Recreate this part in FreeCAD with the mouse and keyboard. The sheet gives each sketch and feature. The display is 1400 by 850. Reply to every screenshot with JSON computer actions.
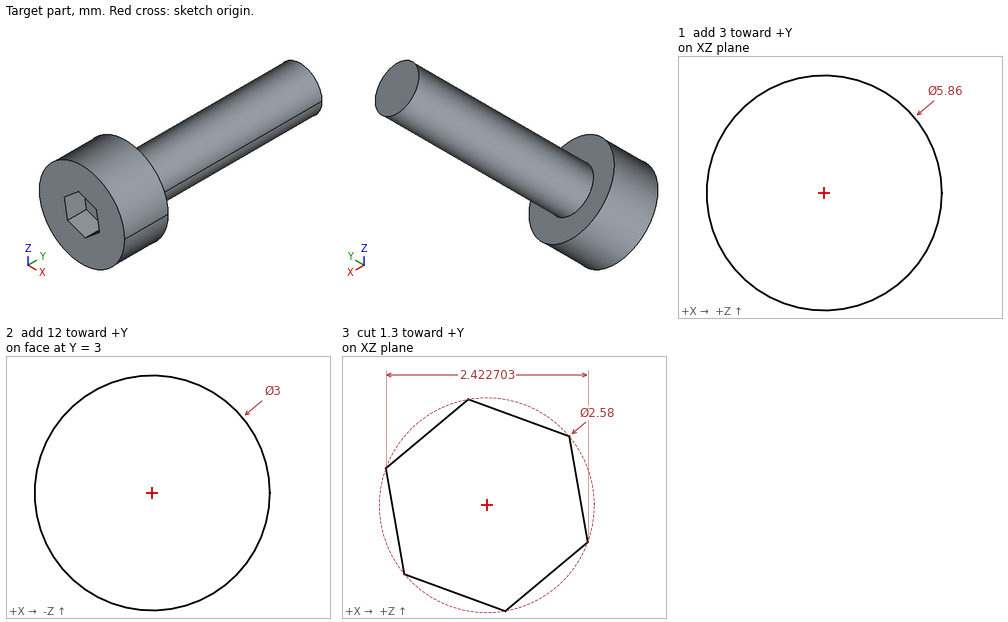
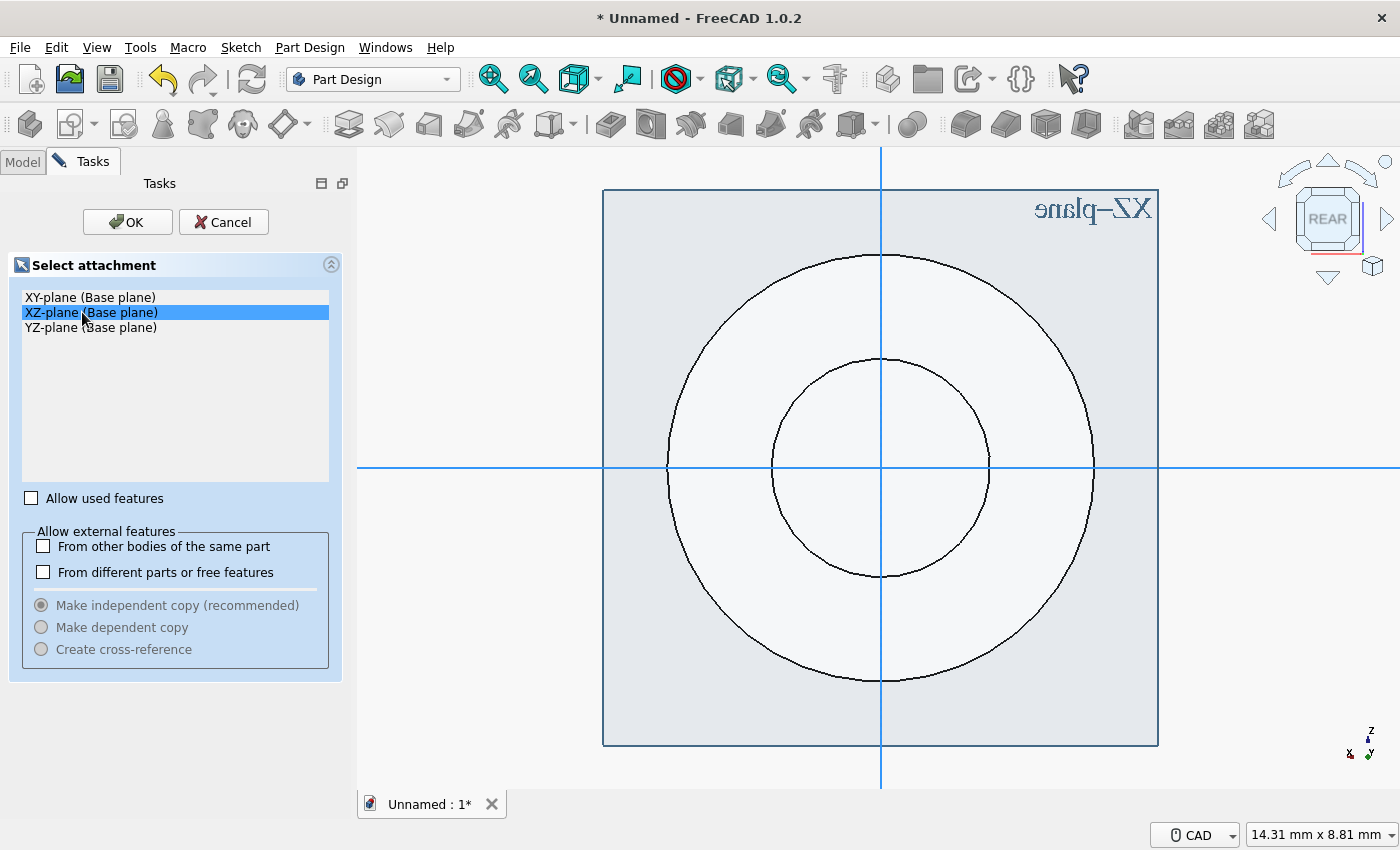
{"action": "left_click", "coordinate": [128, 222]}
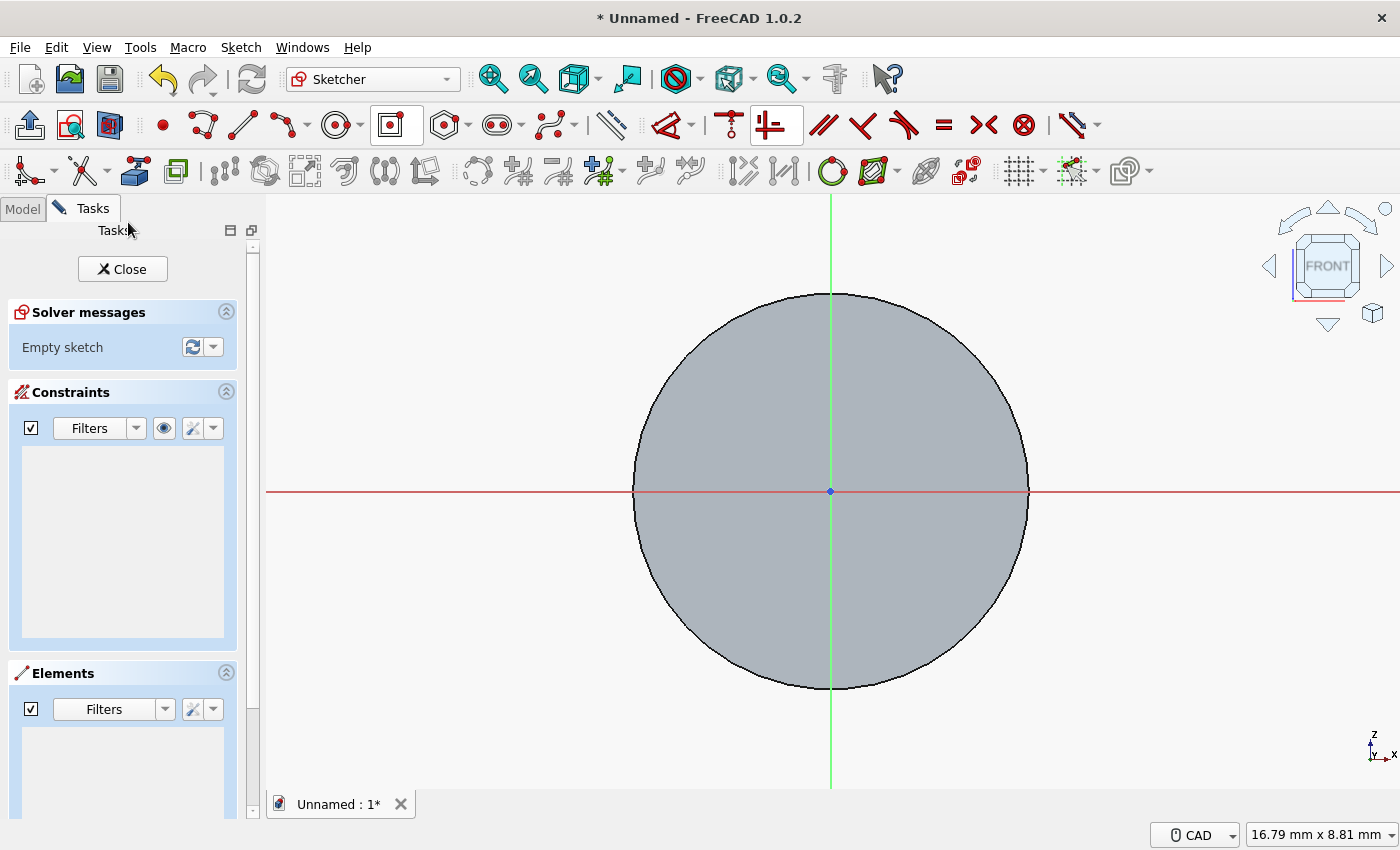
{"action": "scroll", "coordinate": [885, 491], "scroll_direction": "up", "scroll_amount": 4}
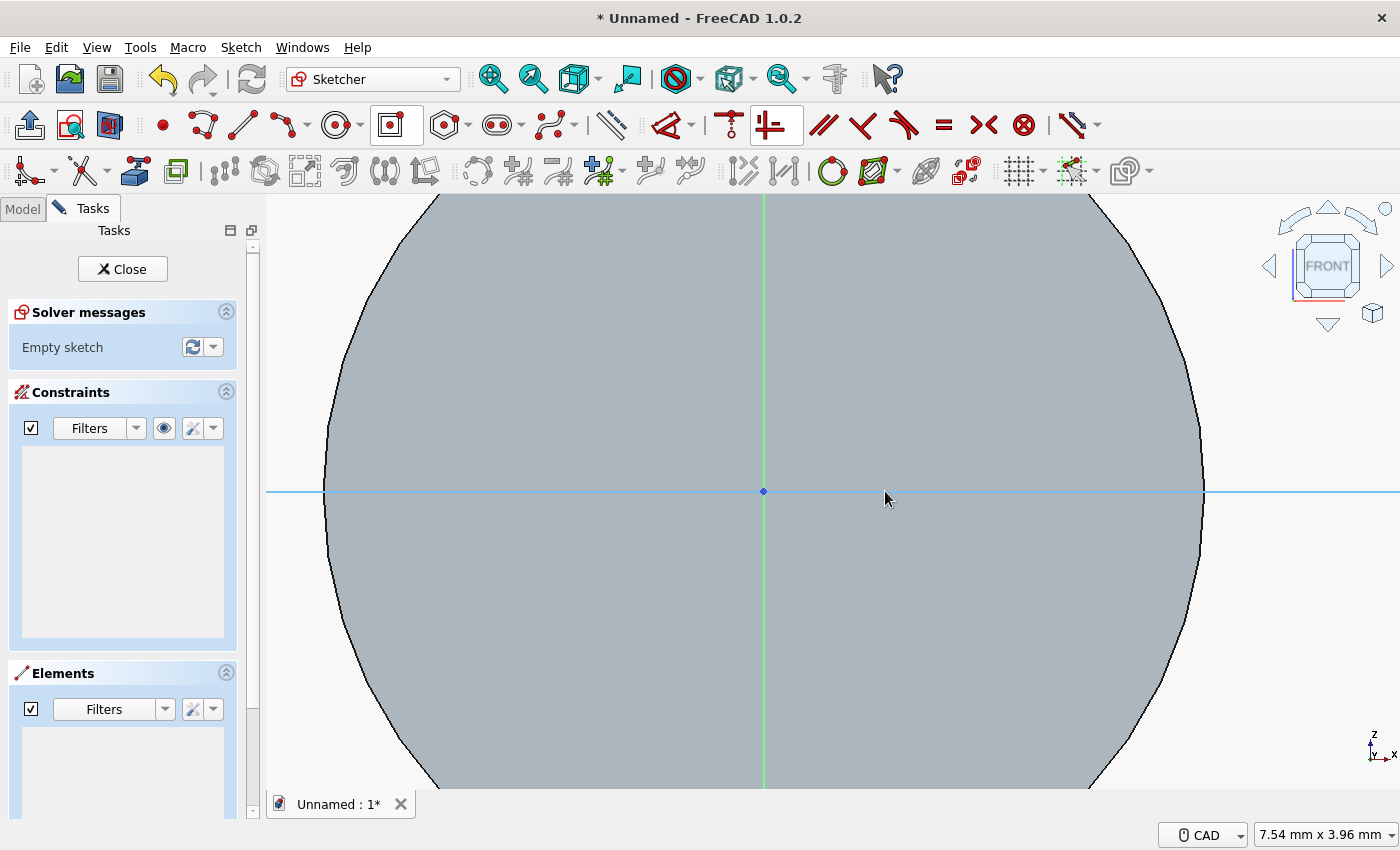
{"action": "left_click", "coordinate": [444, 126]}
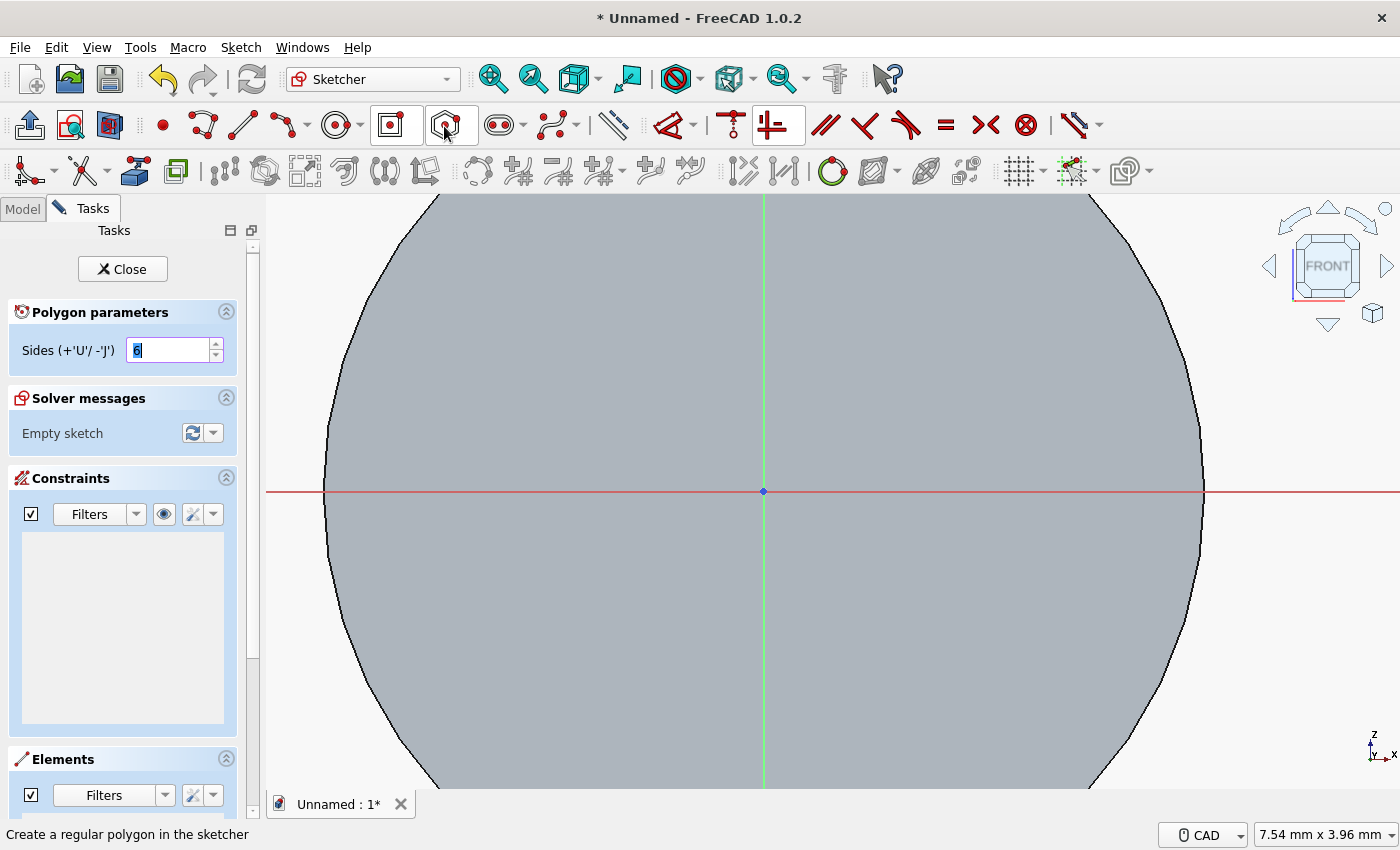
{"action": "left_click", "coordinate": [764, 491]}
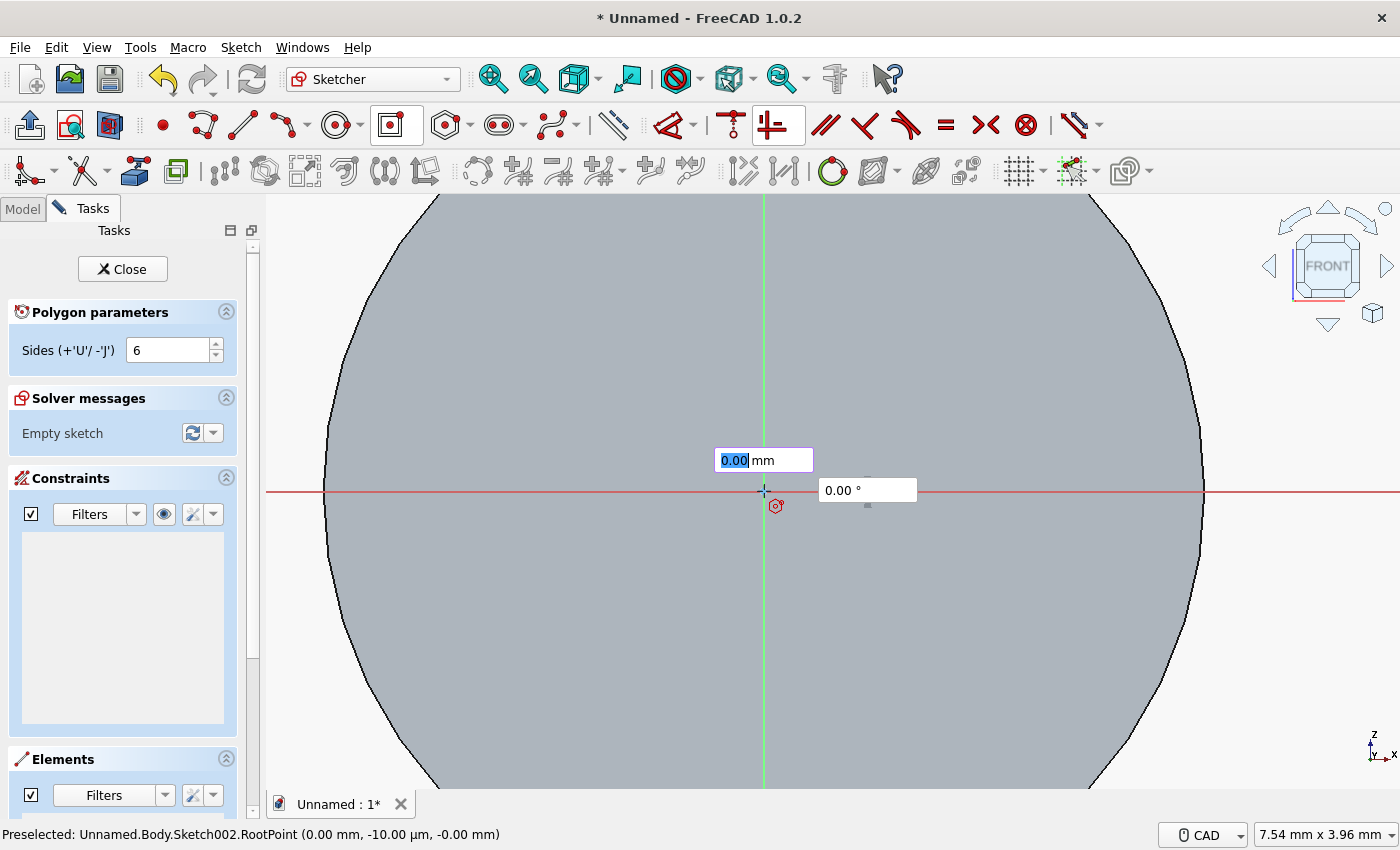
{"action": "left_click", "coordinate": [913, 367]}
{"action": "right_click", "coordinate": [913, 367]}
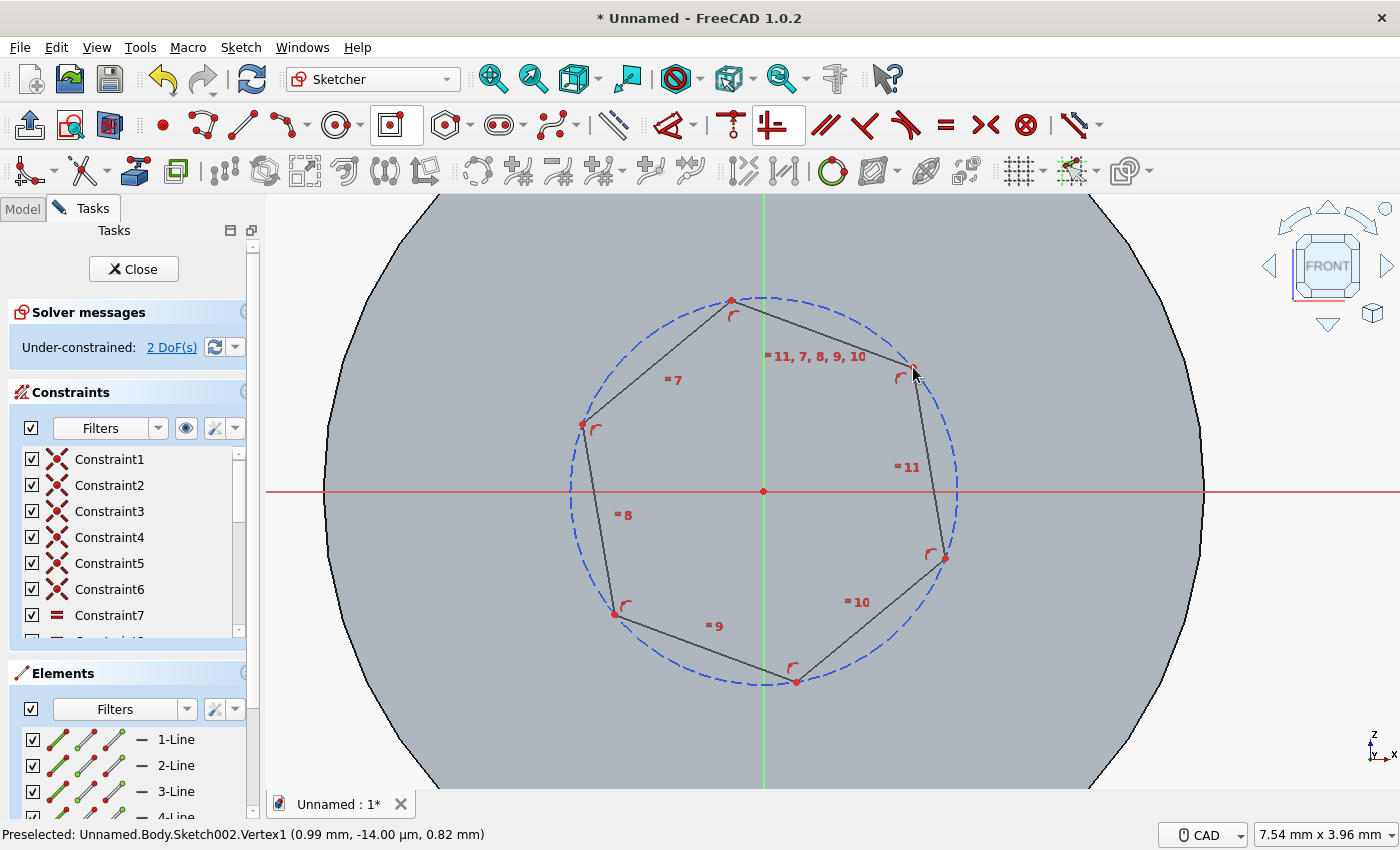
{"action": "left_click", "coordinate": [668, 126]}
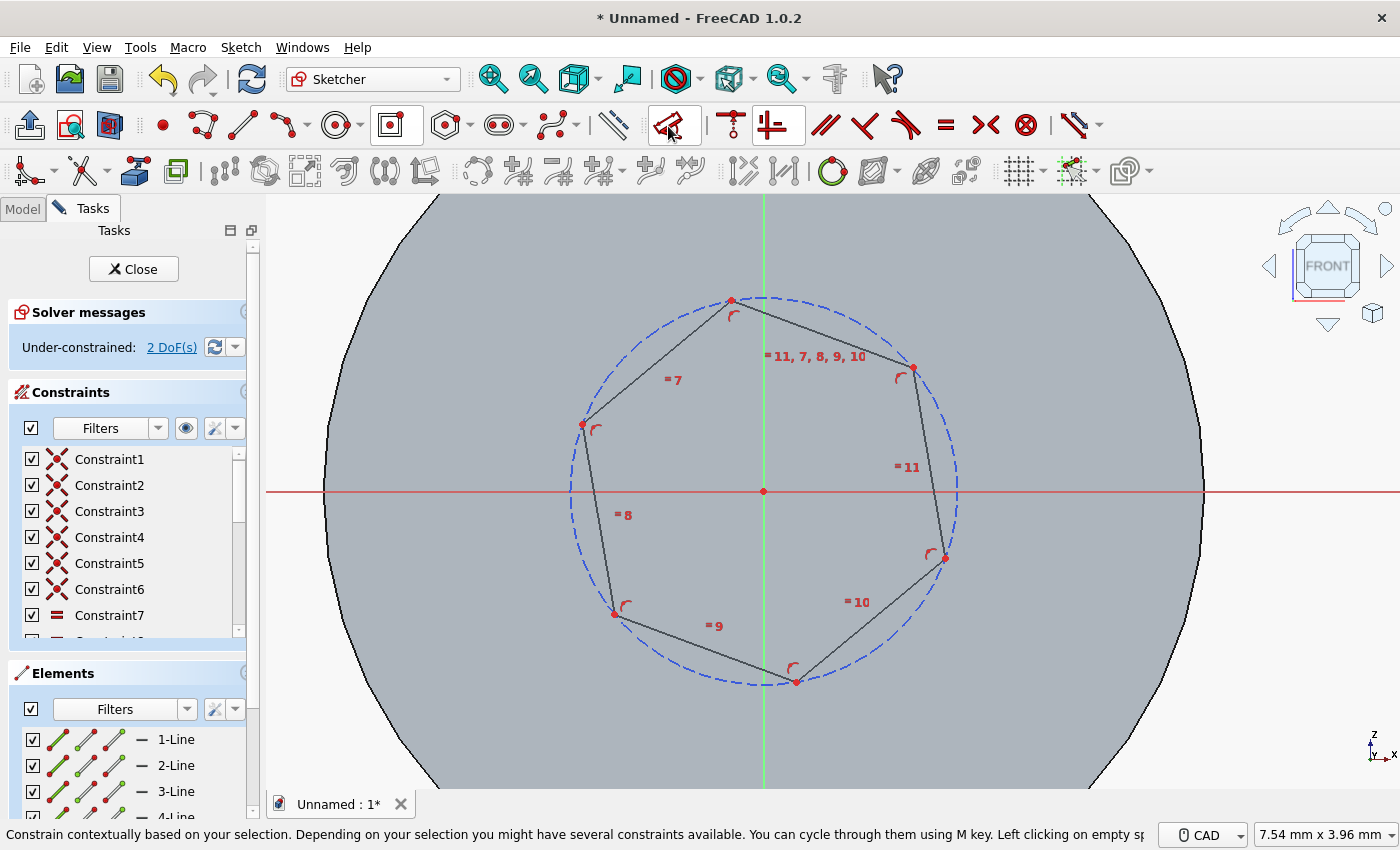
{"action": "left_click", "coordinate": [627, 355]}
{"action": "left_click", "coordinate": [604, 332]}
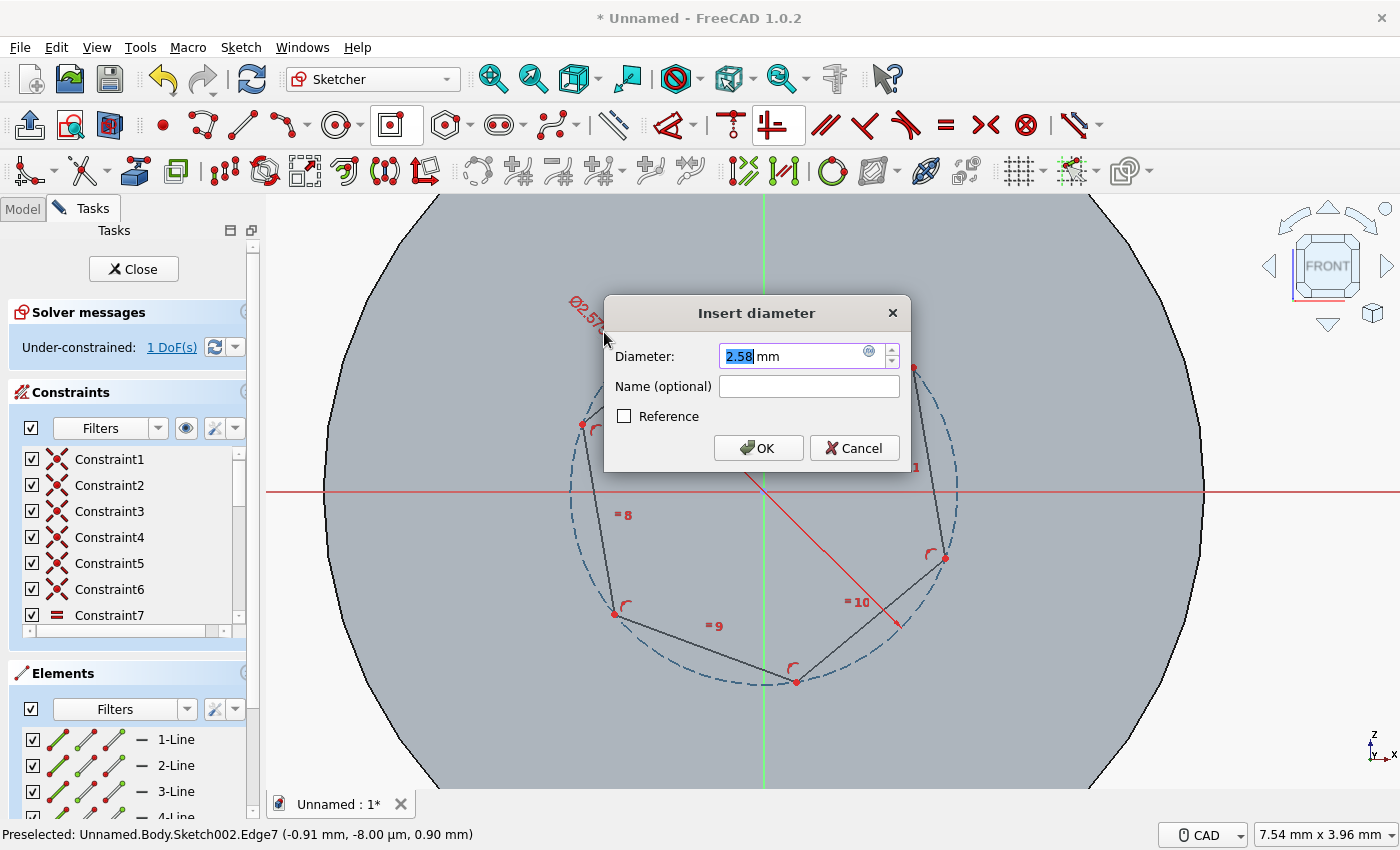
{"action": "type", "text": "2.58"}
{"action": "key", "text": "Return"}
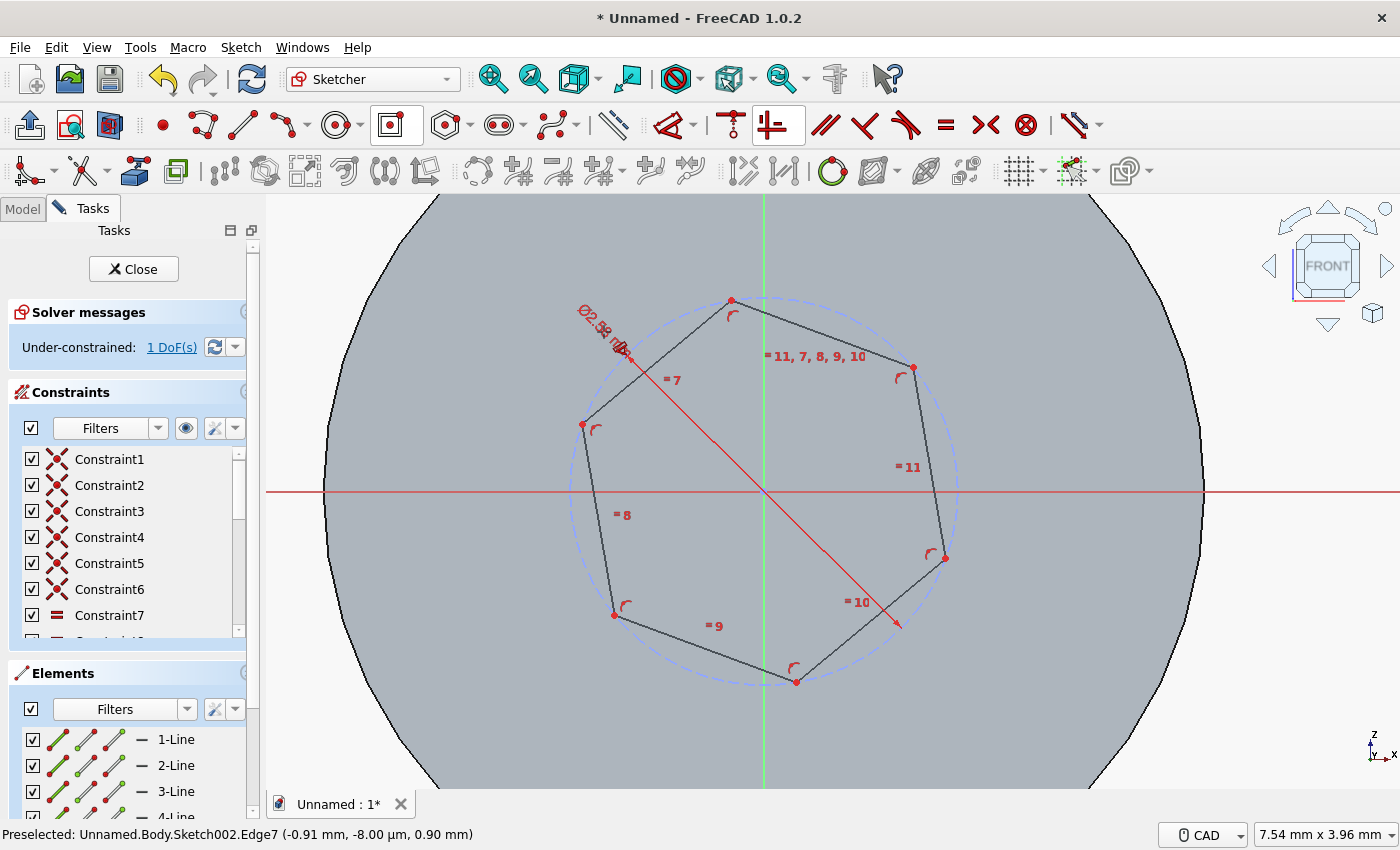
{"action": "left_click", "coordinate": [582, 424]}